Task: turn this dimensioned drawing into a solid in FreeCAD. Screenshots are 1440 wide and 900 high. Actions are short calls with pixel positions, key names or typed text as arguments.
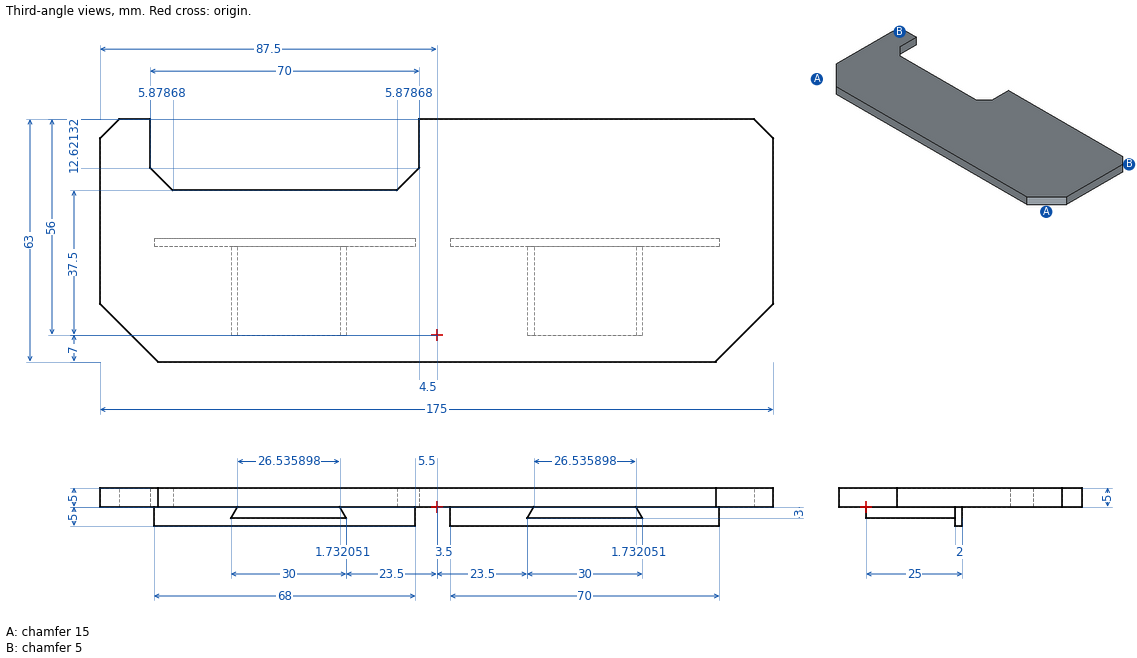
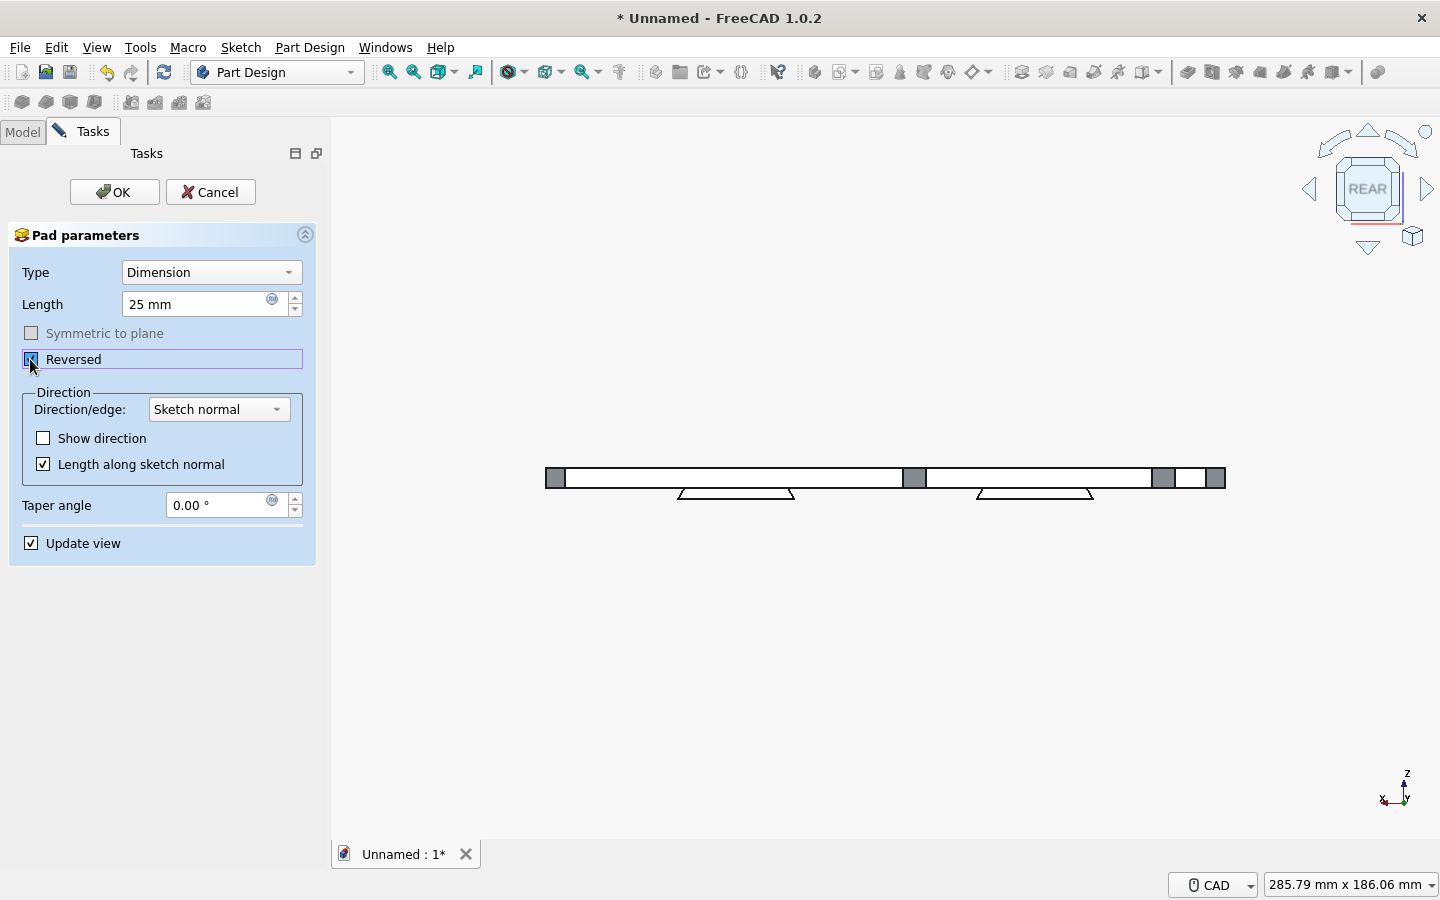
click(115, 192)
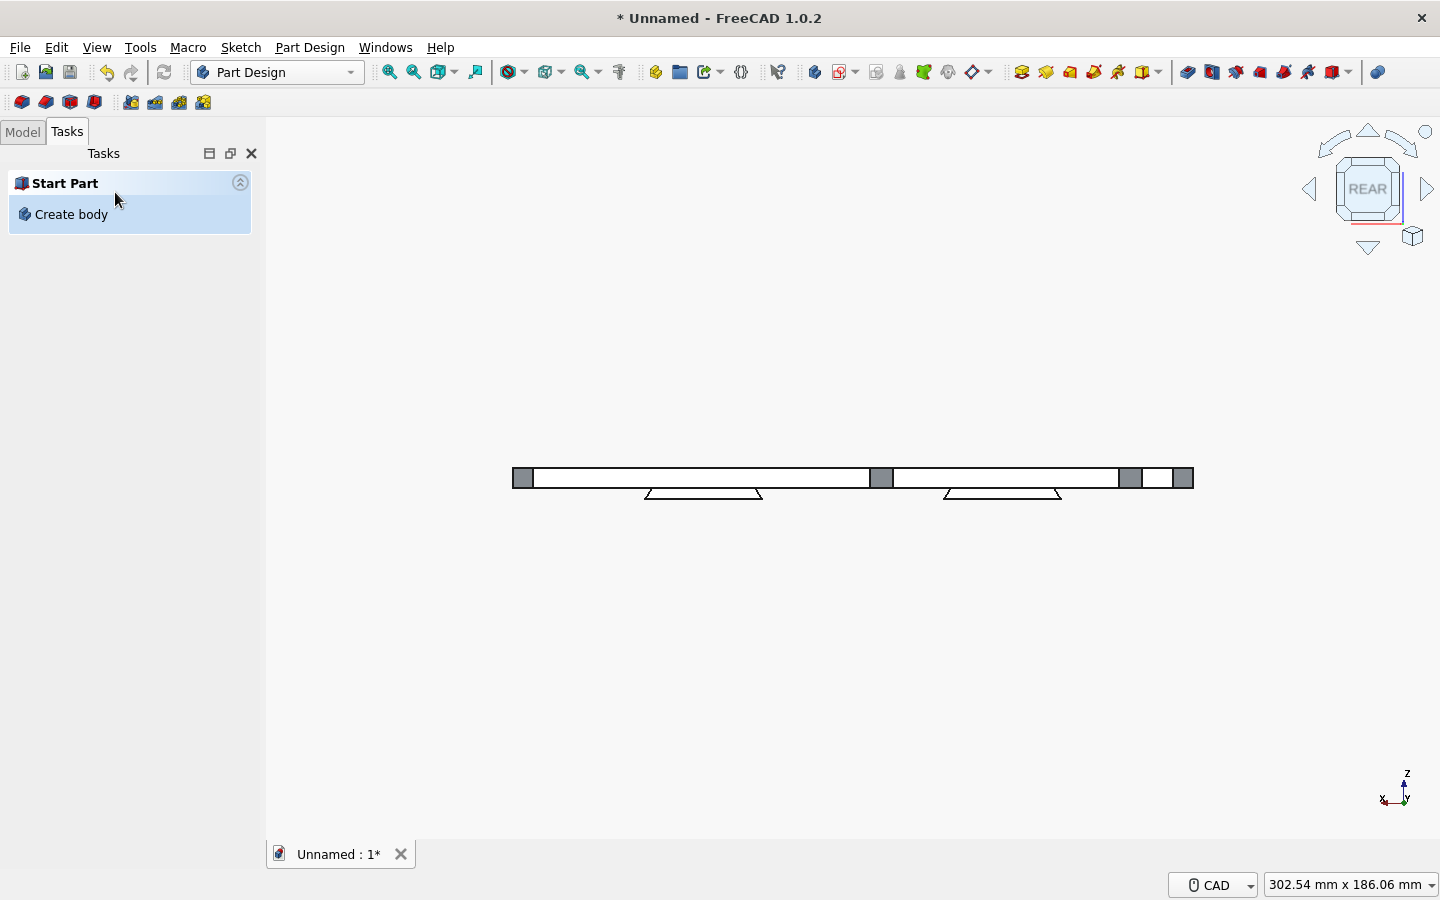
scroll(670, 493, up, 4)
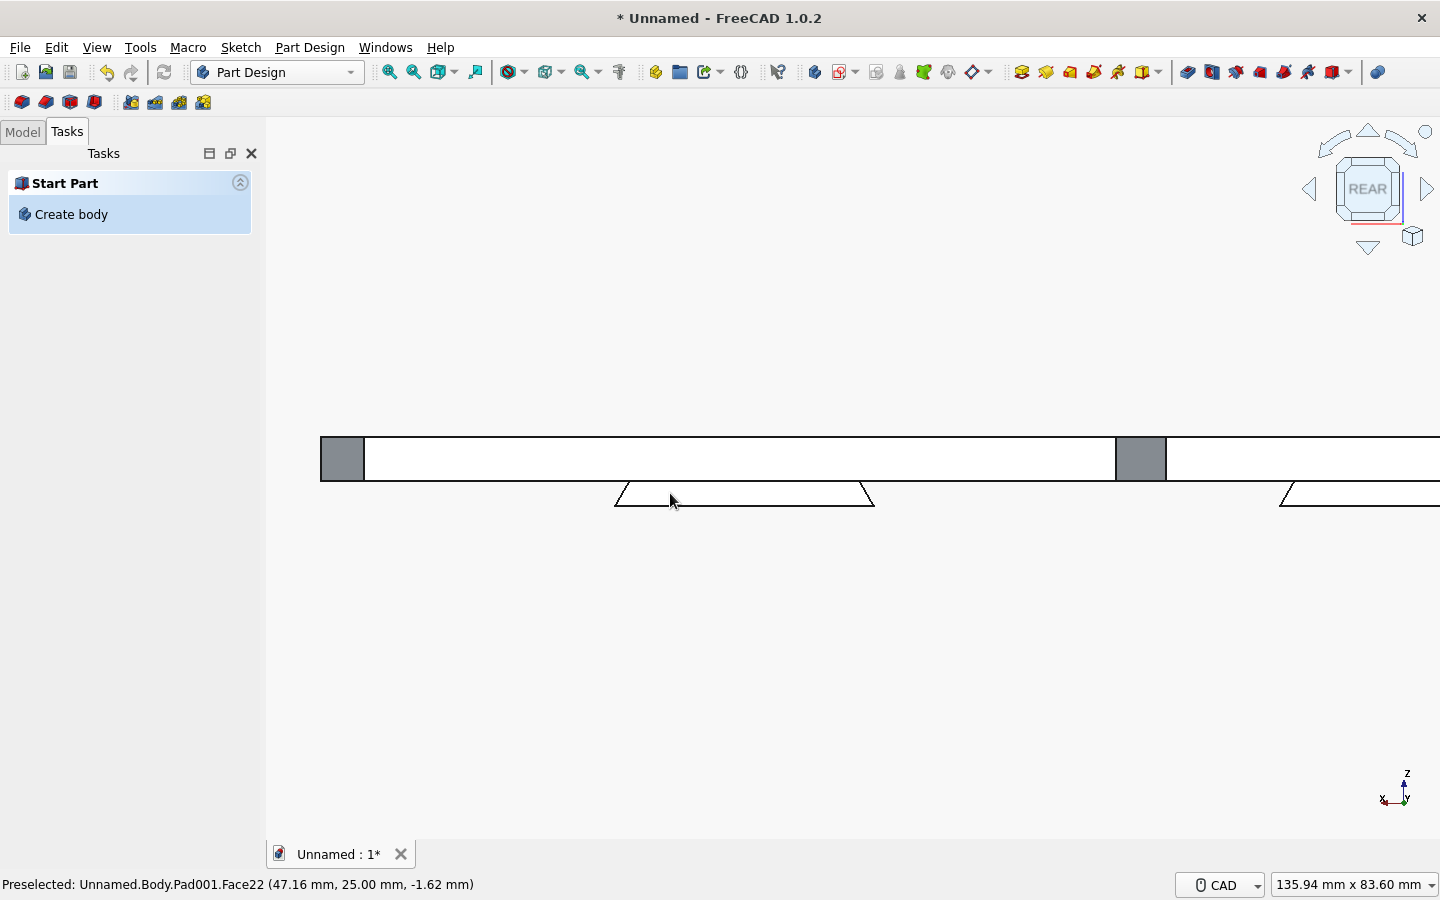
click(670, 493)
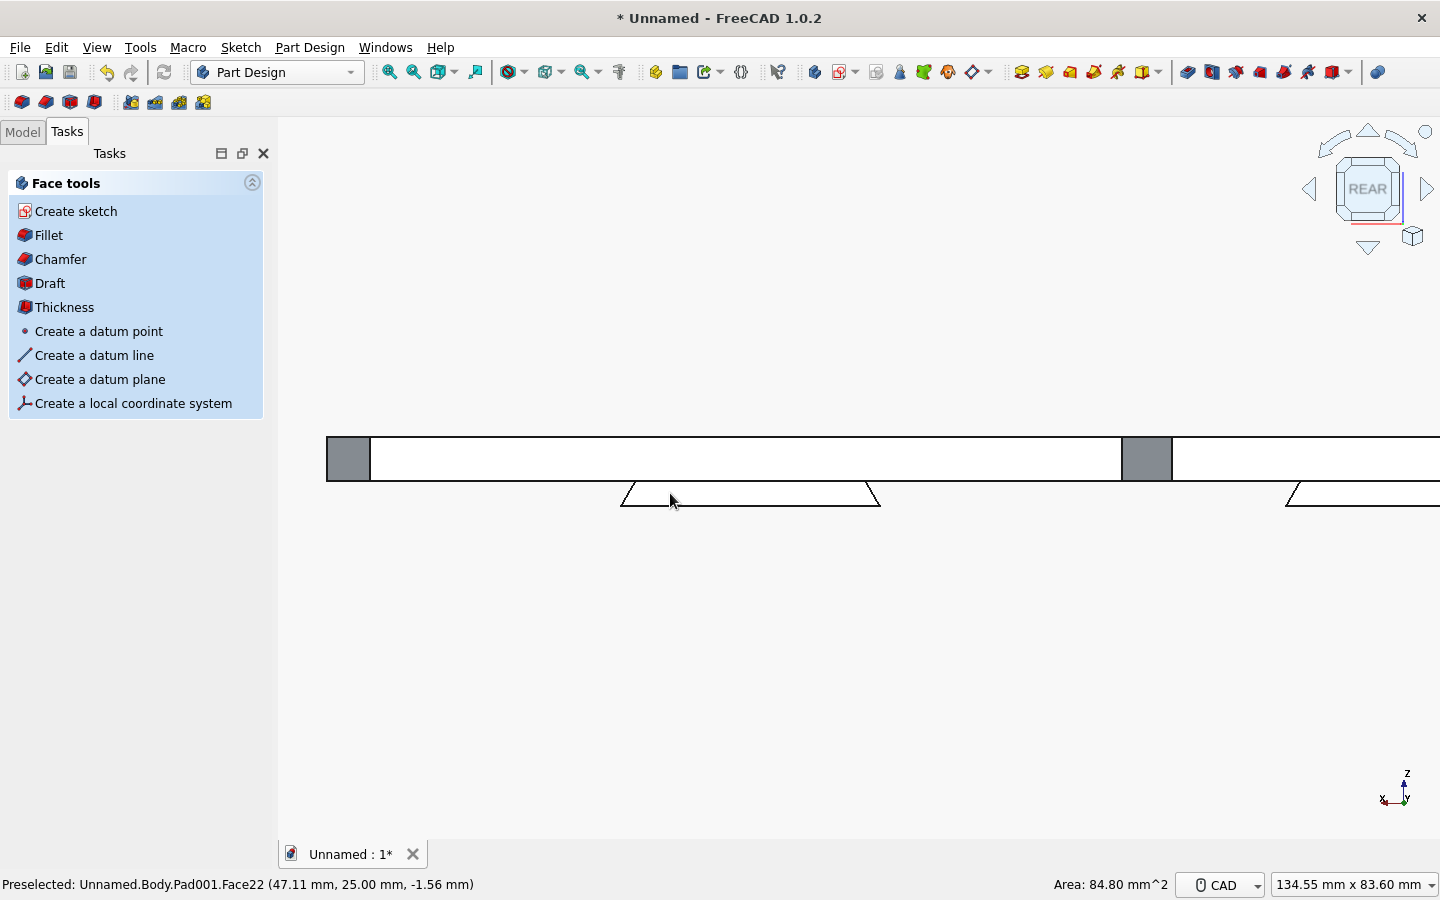
click(840, 72)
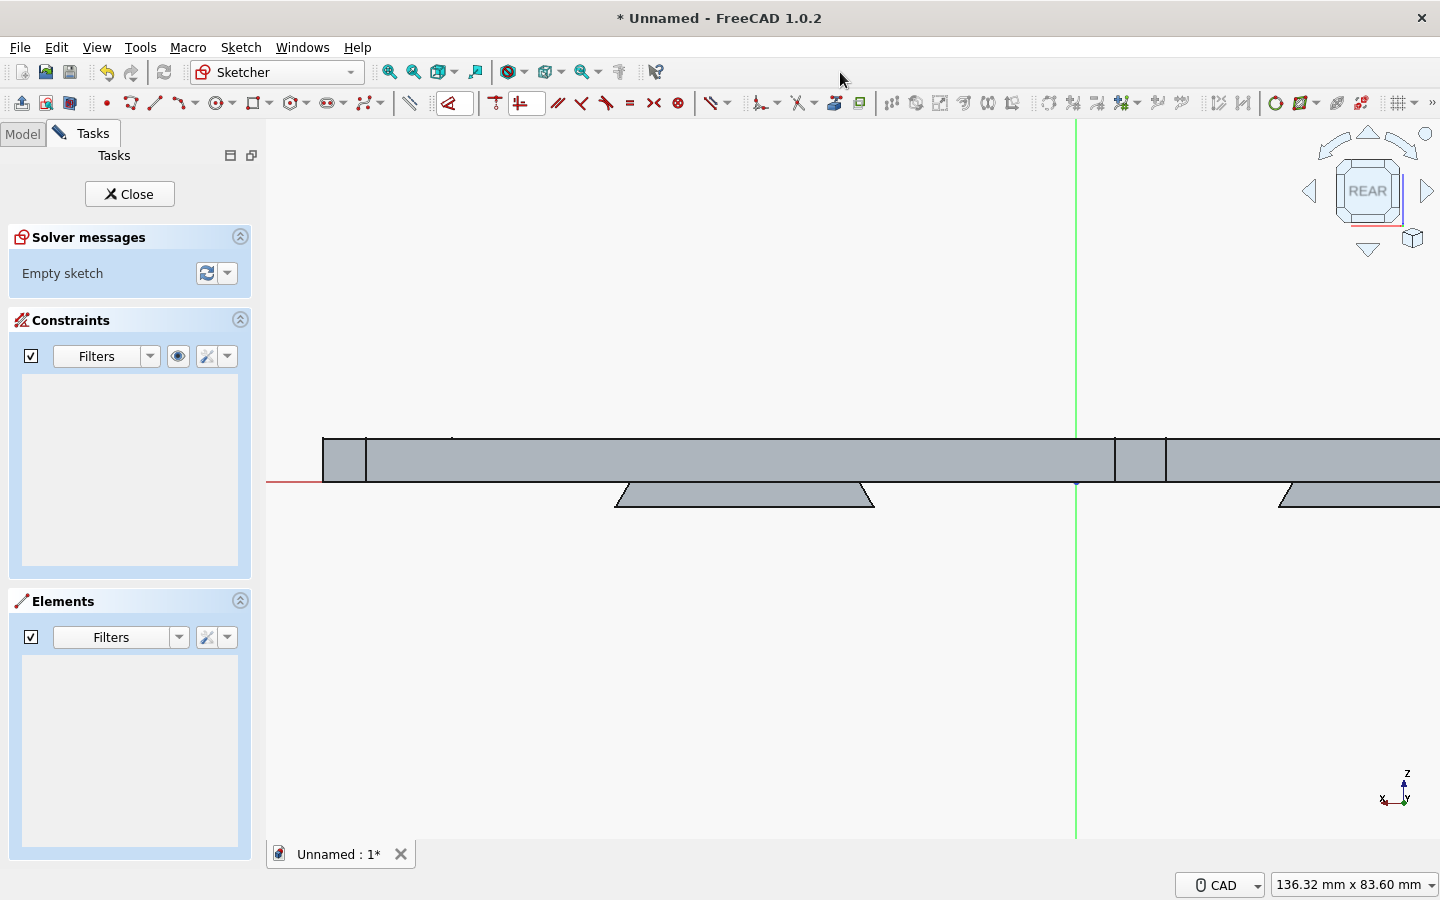
click(70, 104)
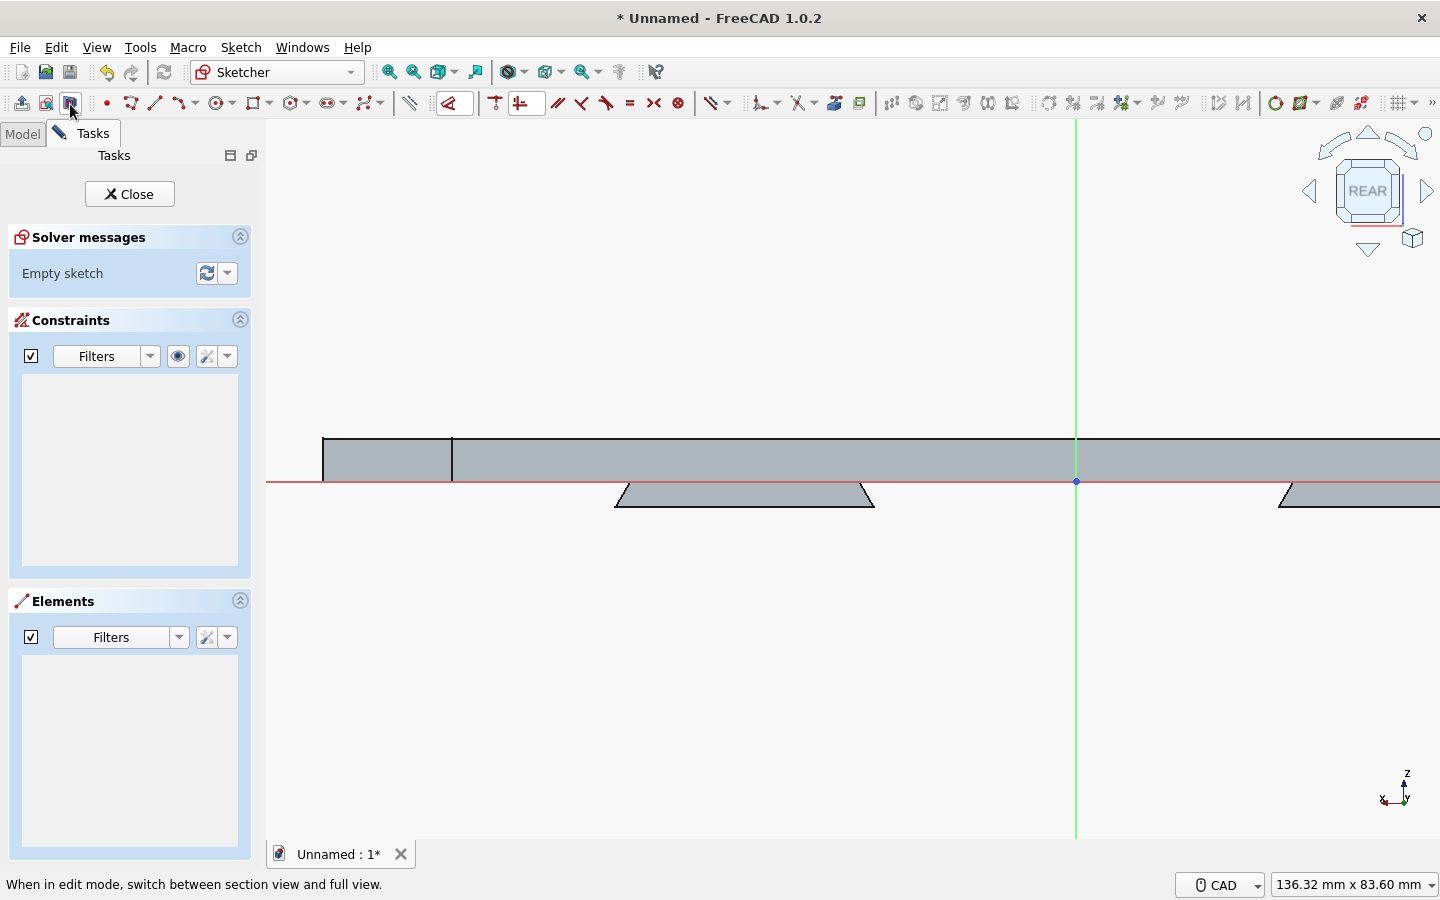
scroll(430, 450, down, 3)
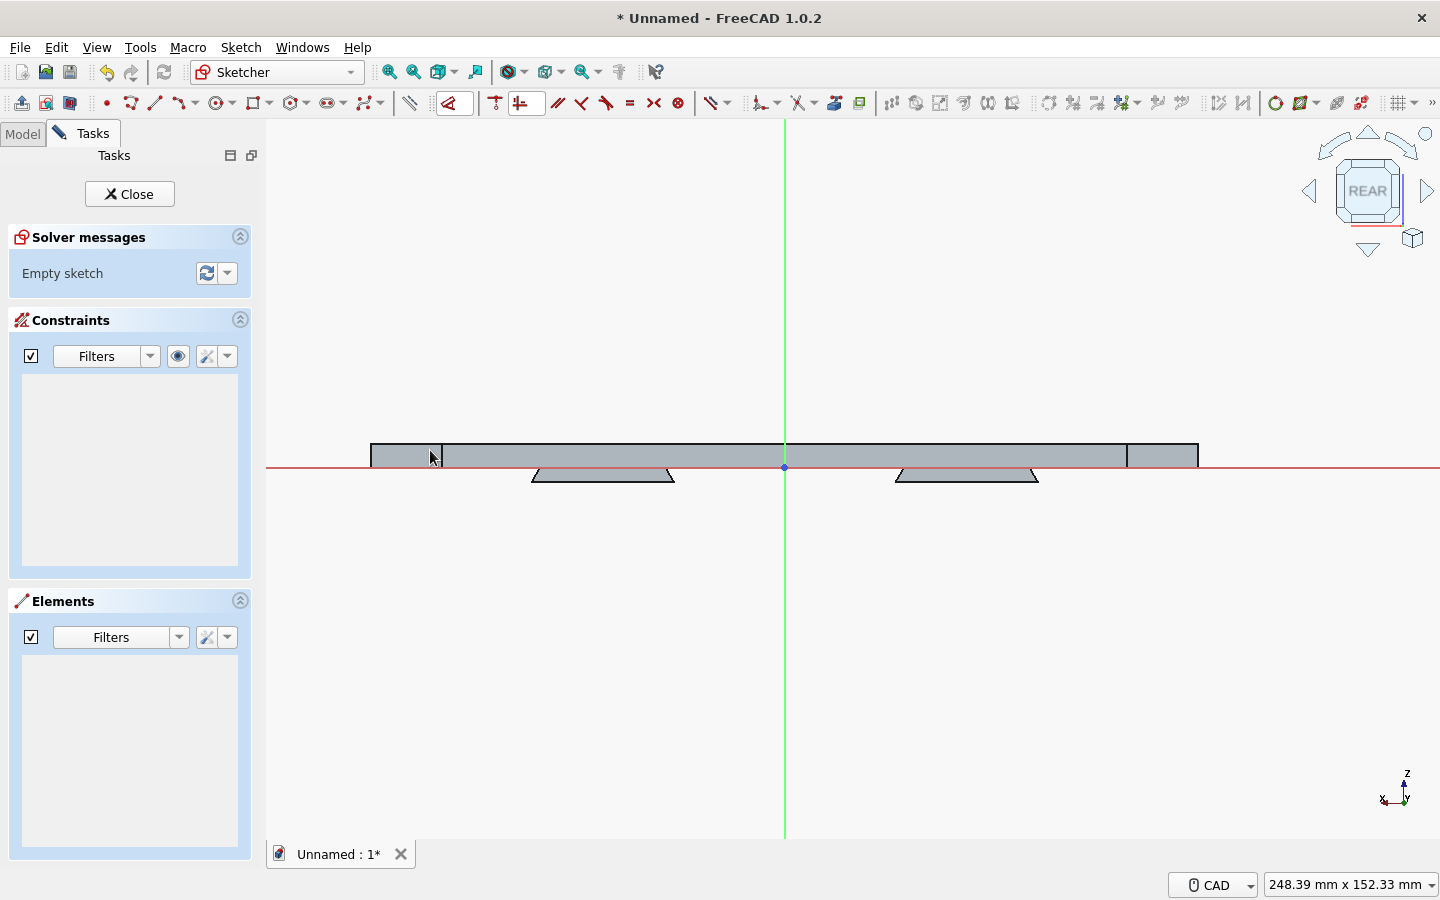
click(254, 104)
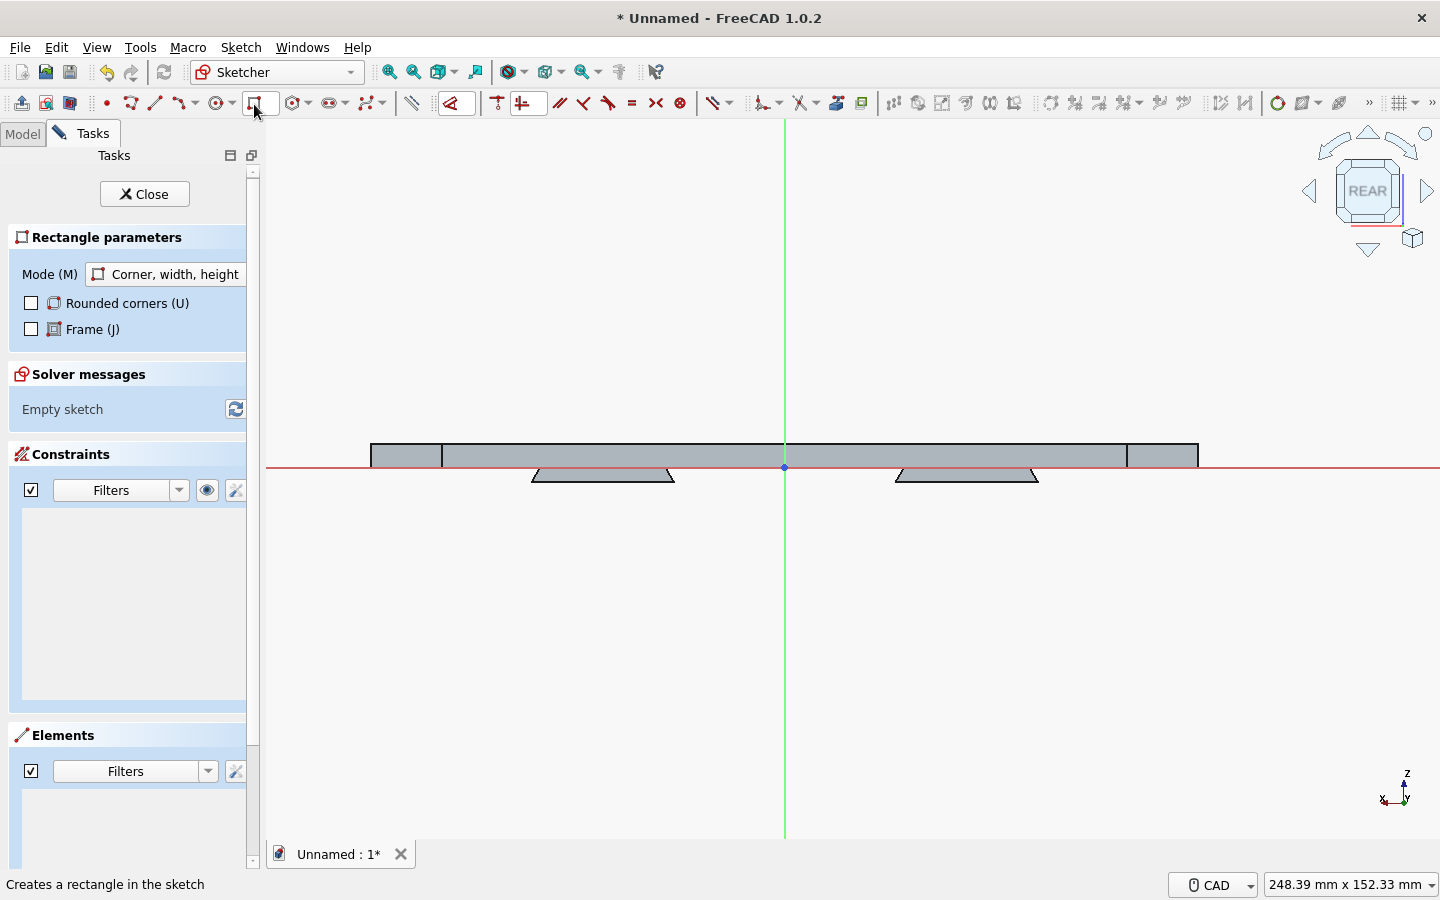
click(811, 468)
click(1132, 491)